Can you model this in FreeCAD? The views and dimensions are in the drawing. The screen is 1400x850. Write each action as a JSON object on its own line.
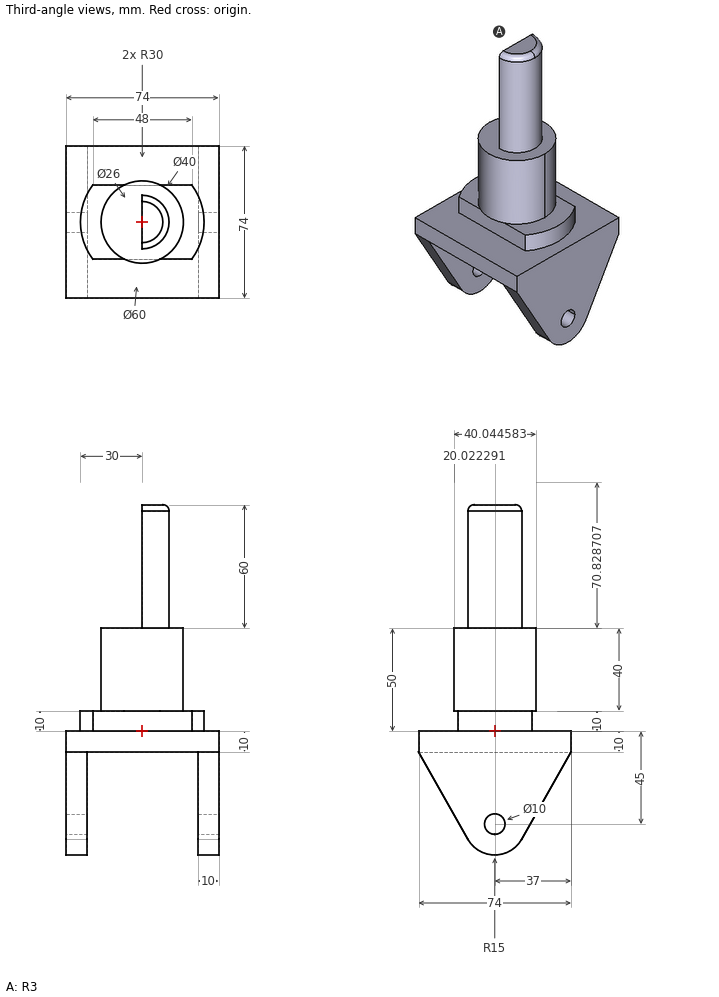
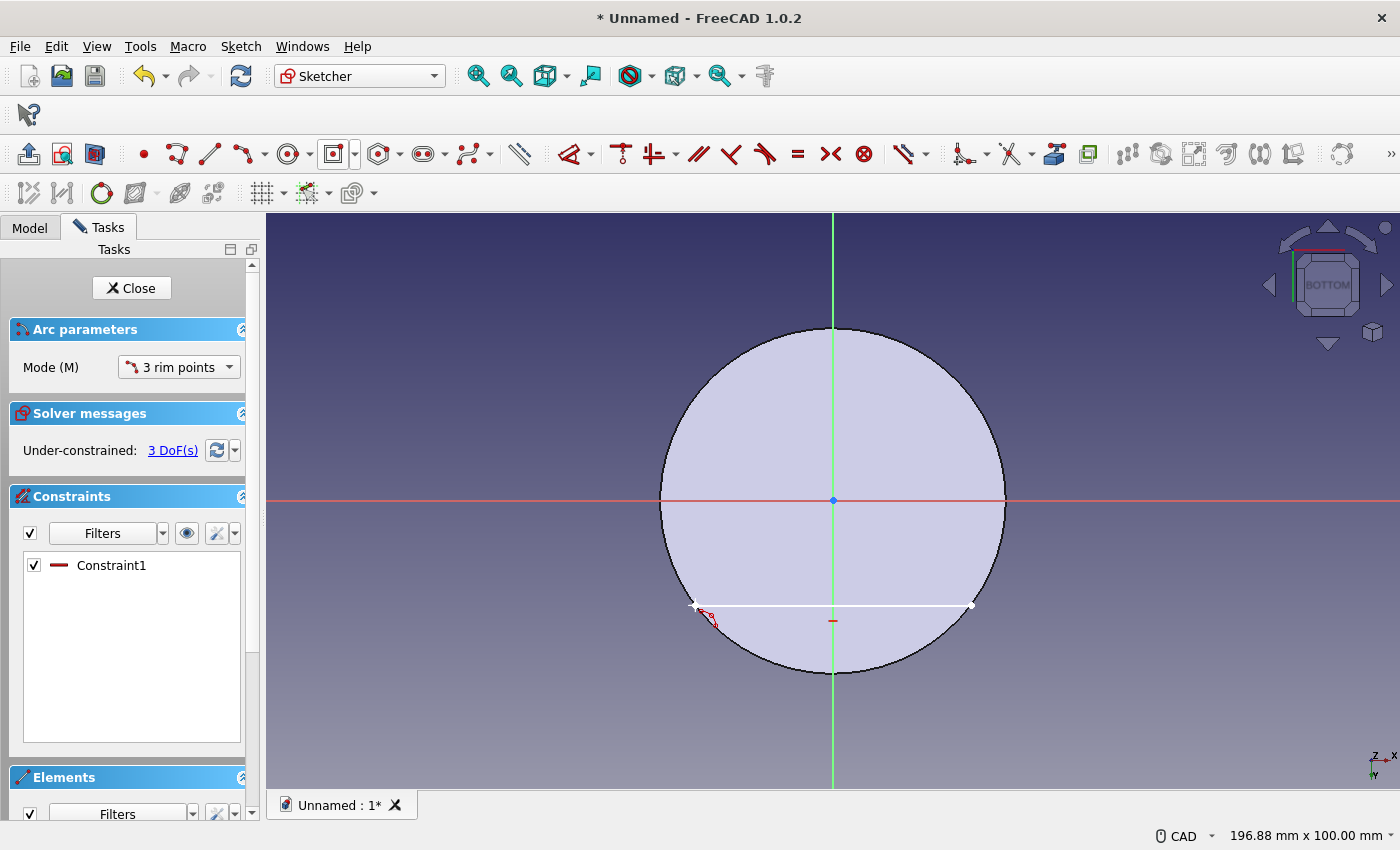
{"action": "left_click", "coordinate": [695, 606]}
{"action": "left_click", "coordinate": [971, 606]}
{"action": "left_click", "coordinate": [801, 671]}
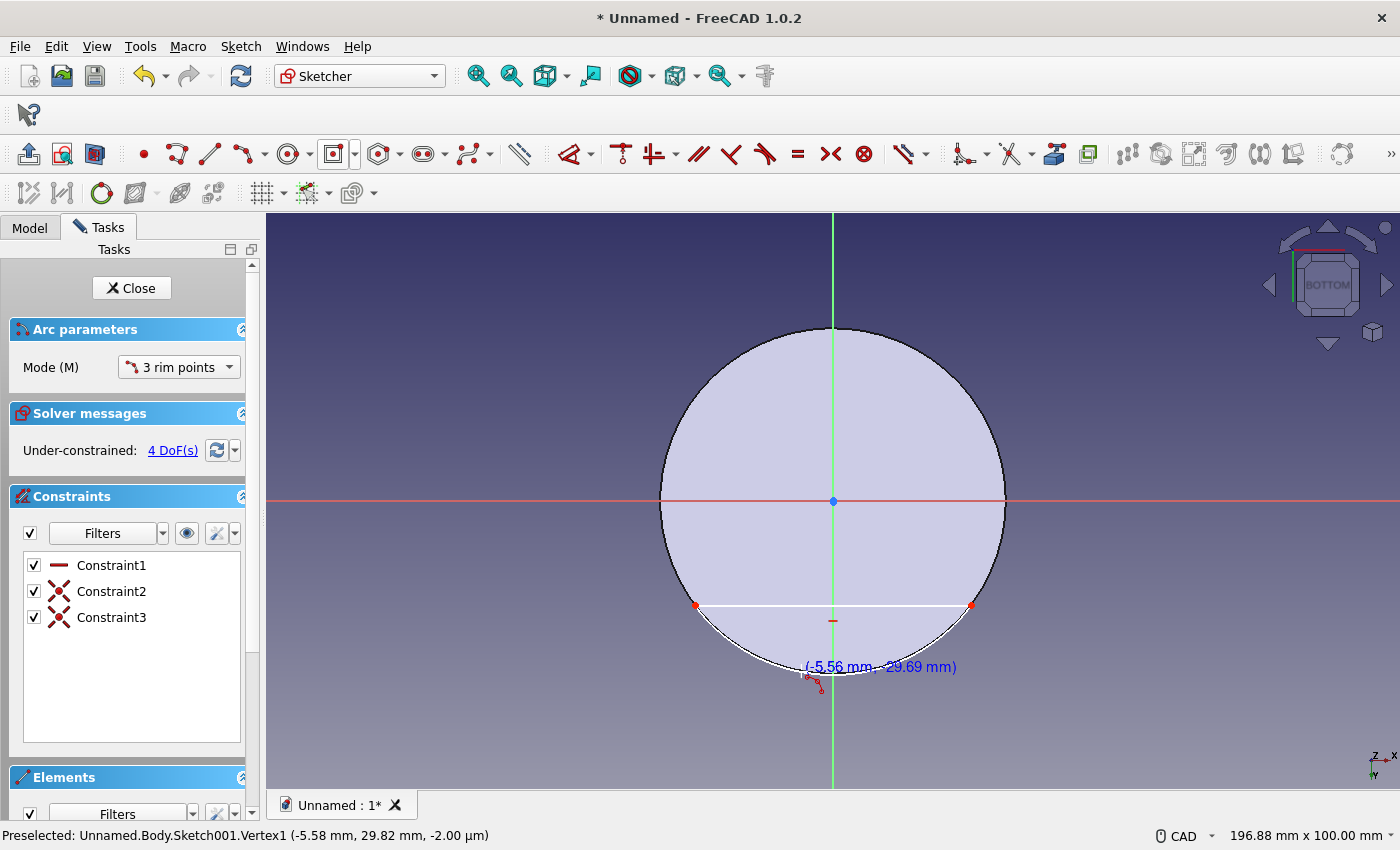
{"action": "key", "text": "g l"}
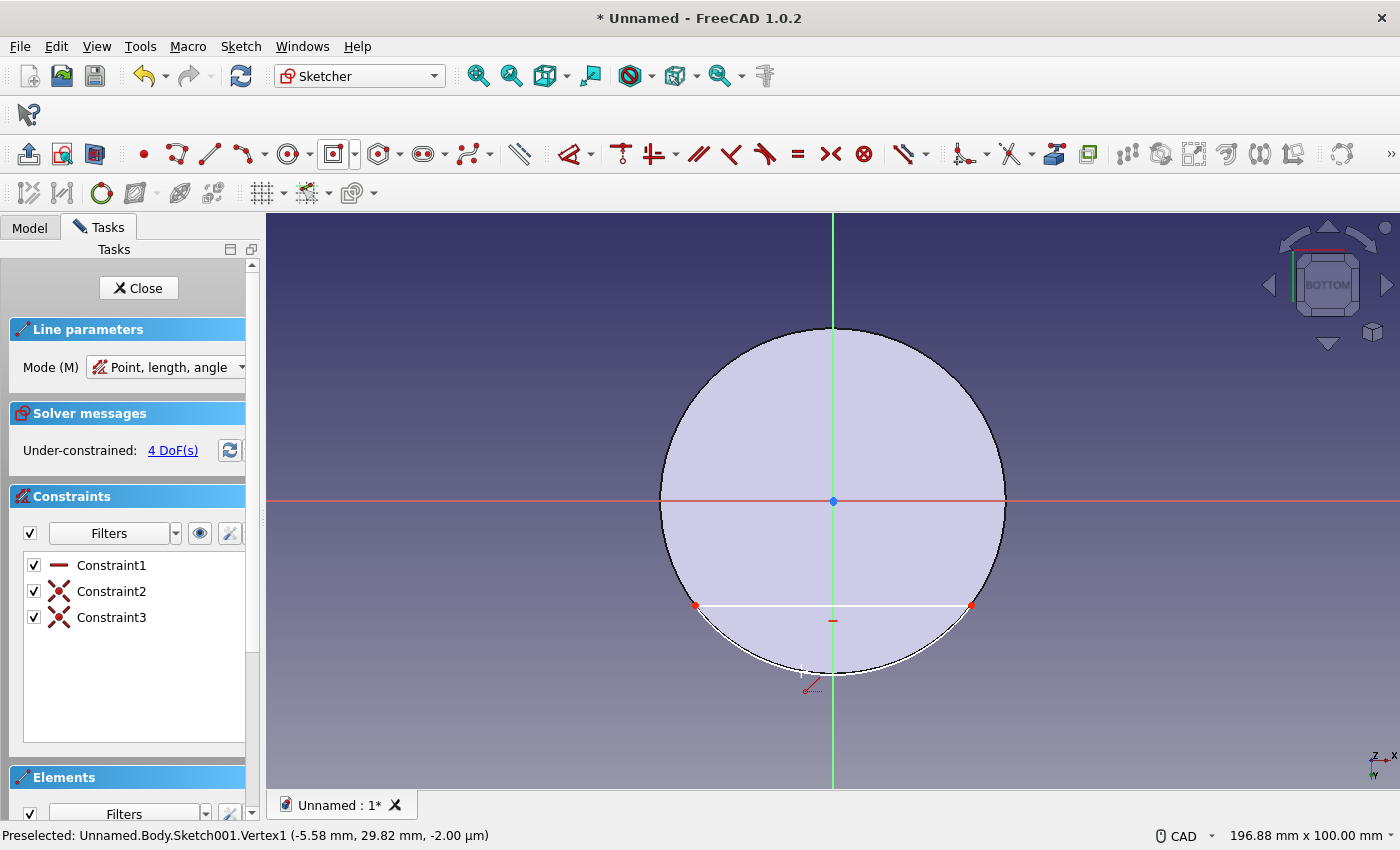
{"action": "left_click", "coordinate": [695, 397]}
{"action": "left_click", "coordinate": [971, 397]}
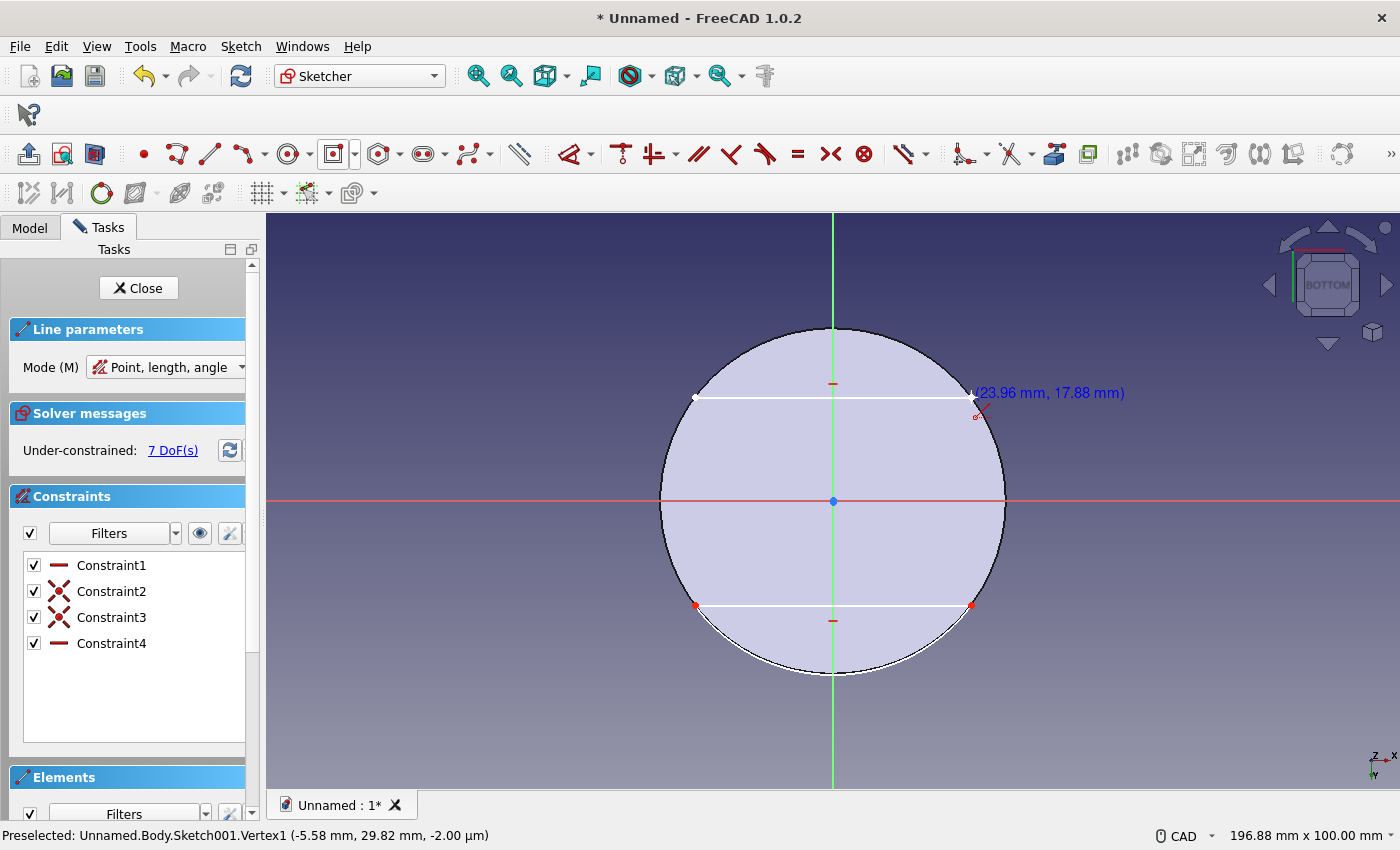
{"action": "key", "text": "g 3 a"}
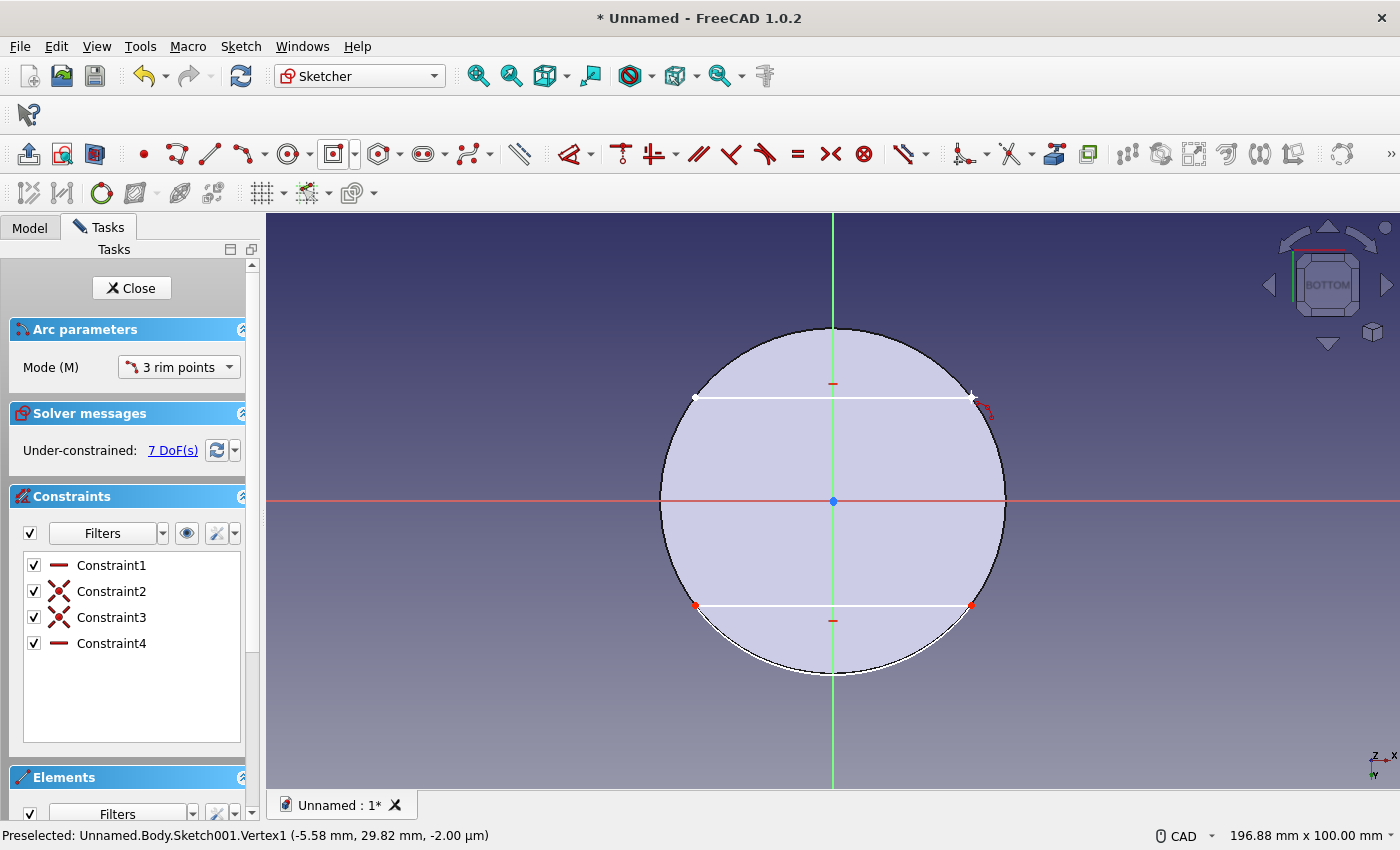
{"action": "left_click", "coordinate": [971, 398]}
{"action": "left_click", "coordinate": [695, 398]}
{"action": "left_click", "coordinate": [865, 331]}
{"action": "key", "text": "Escape"}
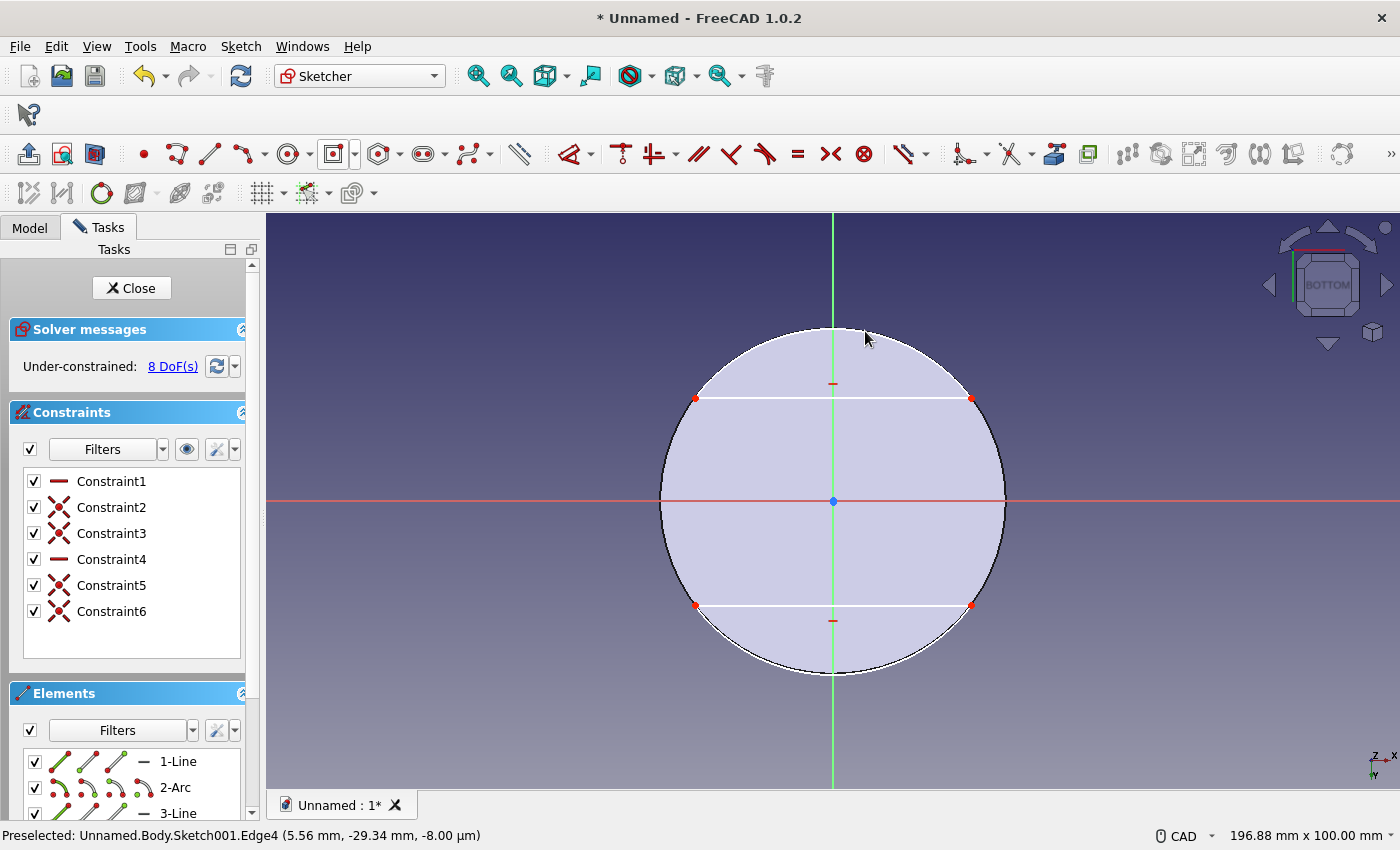
{"action": "left_click", "coordinate": [770, 663]}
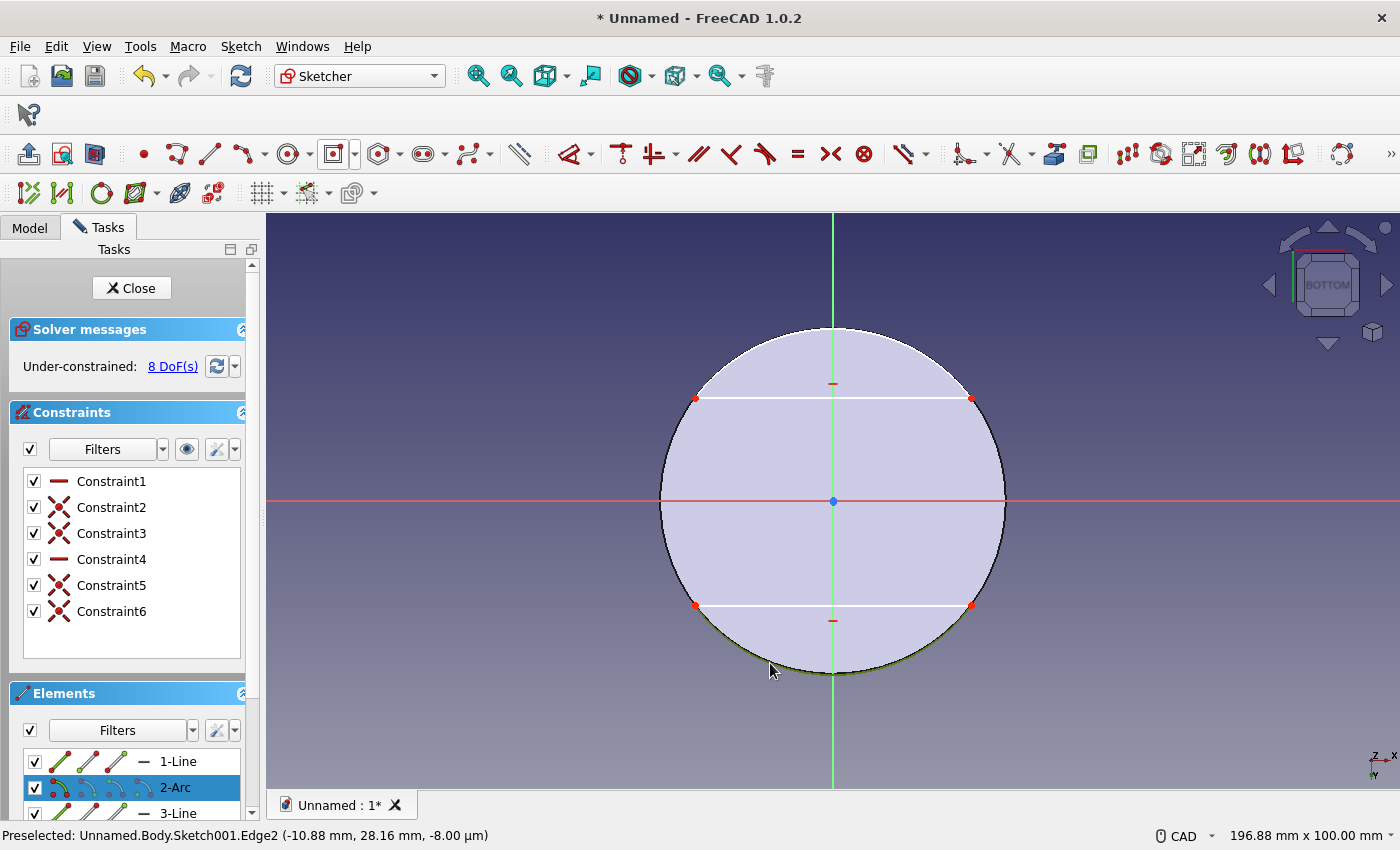
{"action": "left_click", "coordinate": [896, 341]}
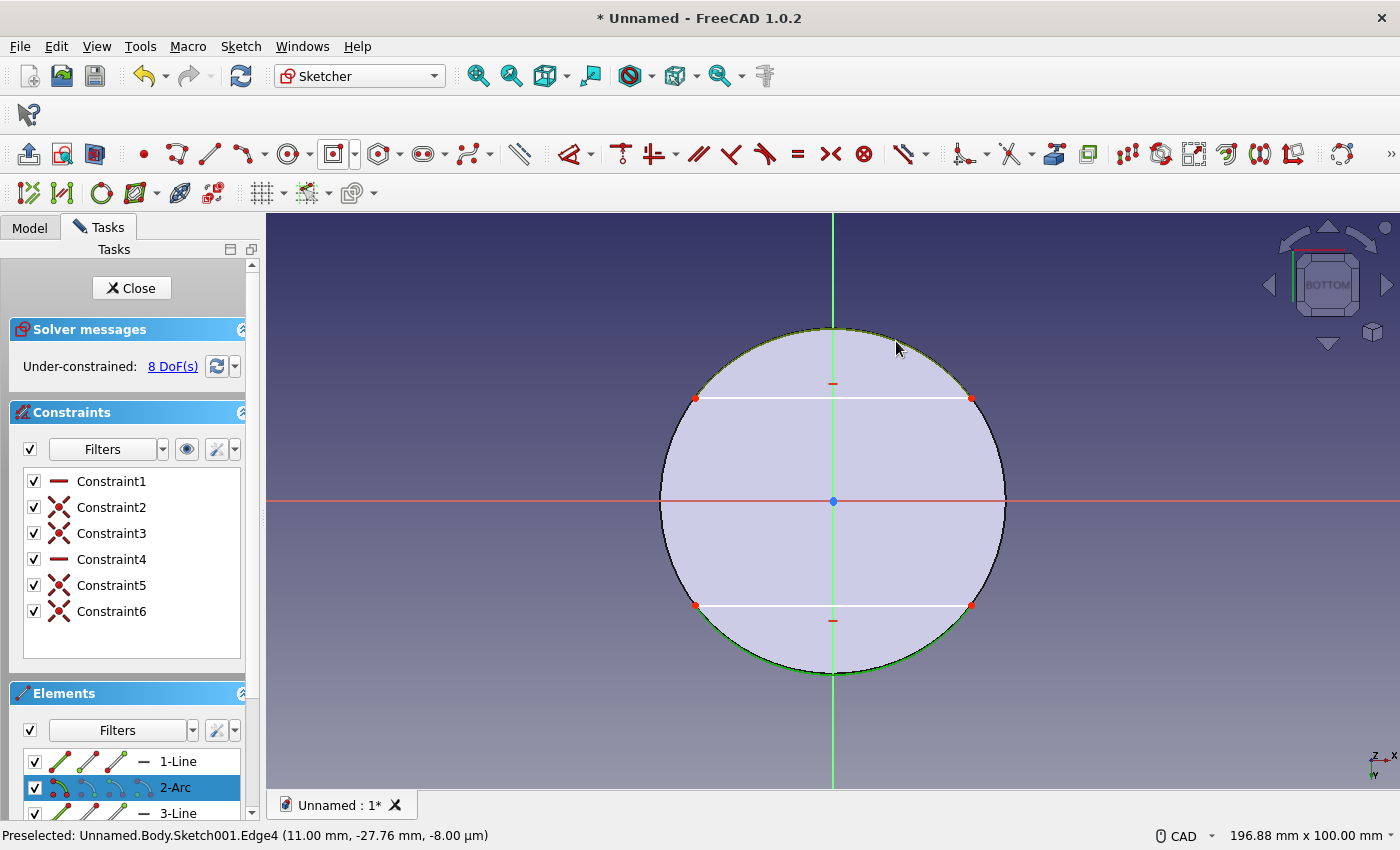
{"action": "left_click", "coordinate": [621, 154]}